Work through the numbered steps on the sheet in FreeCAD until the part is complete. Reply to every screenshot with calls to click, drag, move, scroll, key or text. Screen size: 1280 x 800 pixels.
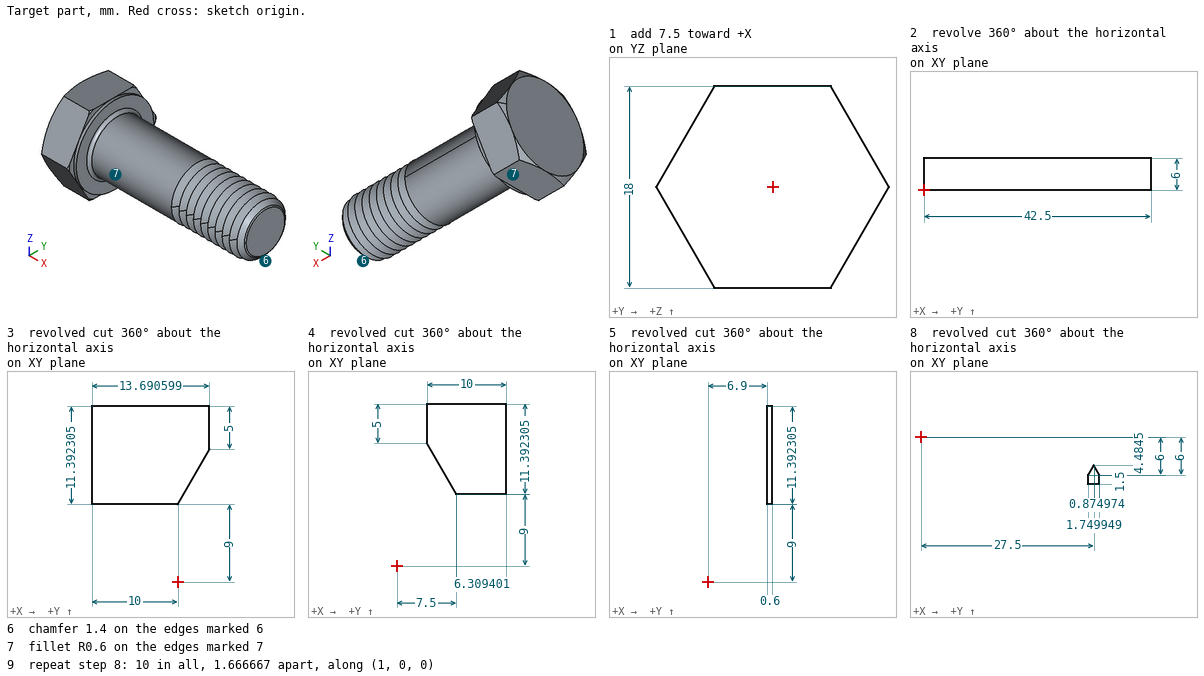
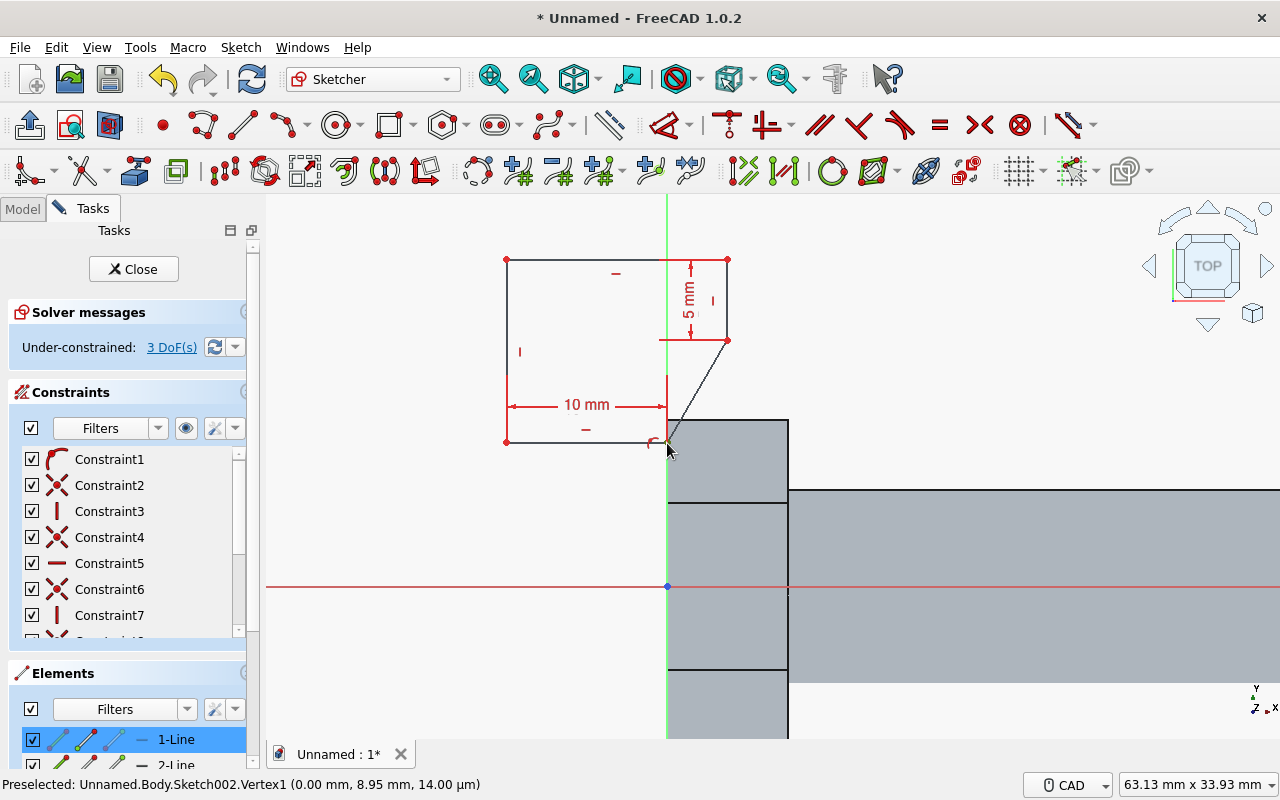
key(i)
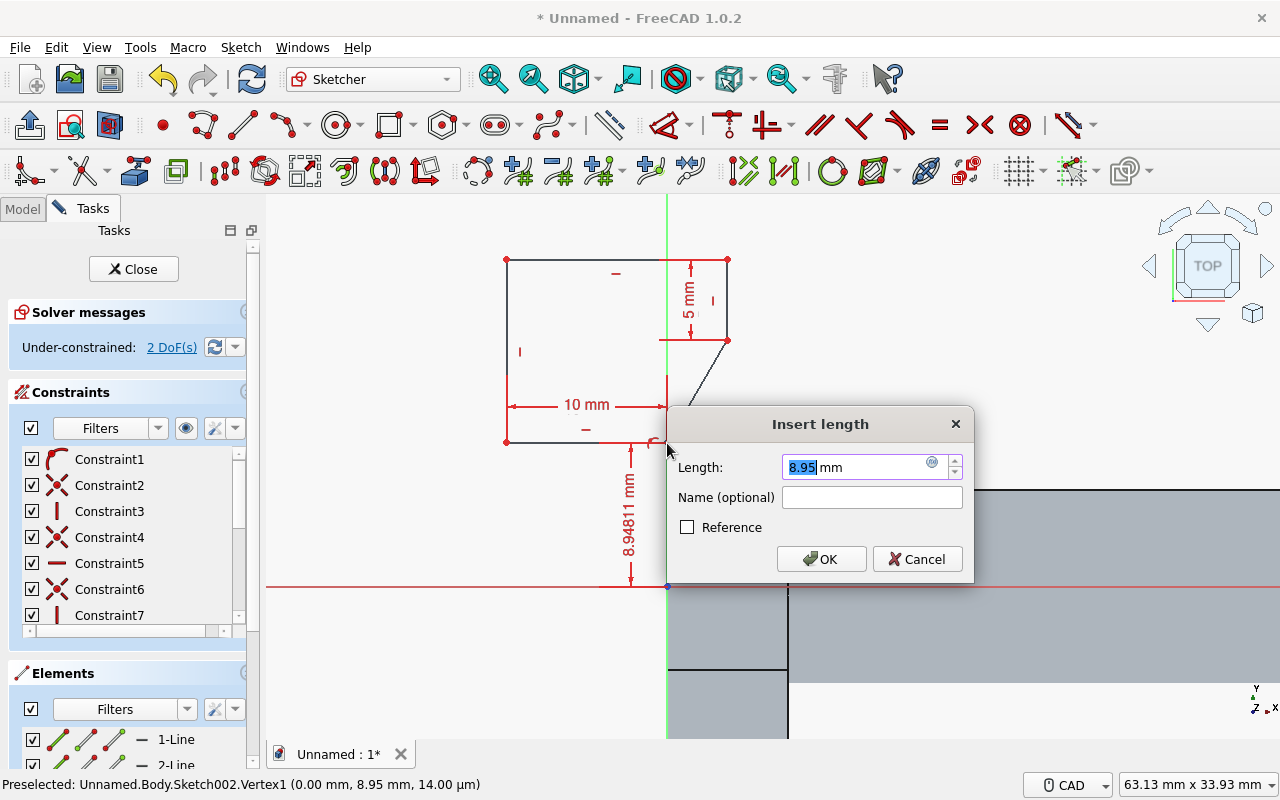
text(9)
key(Return)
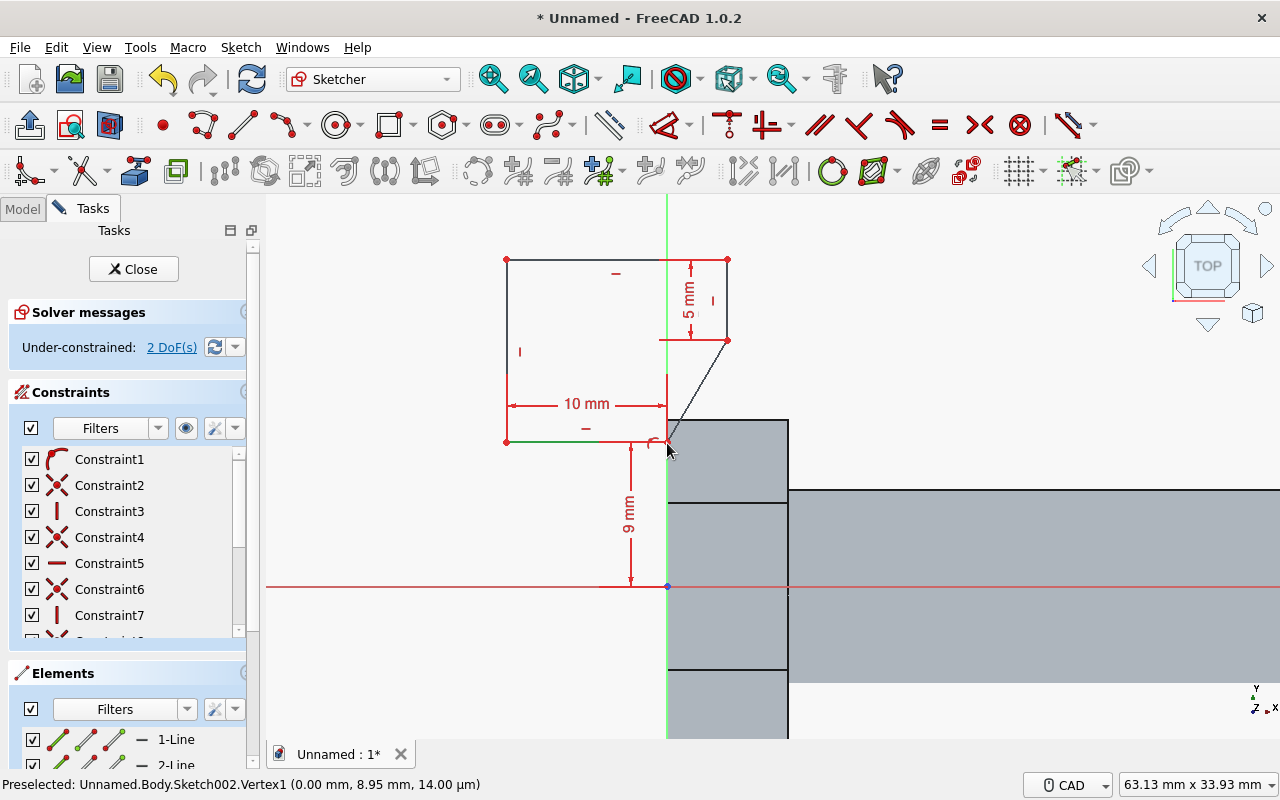
click(573, 260)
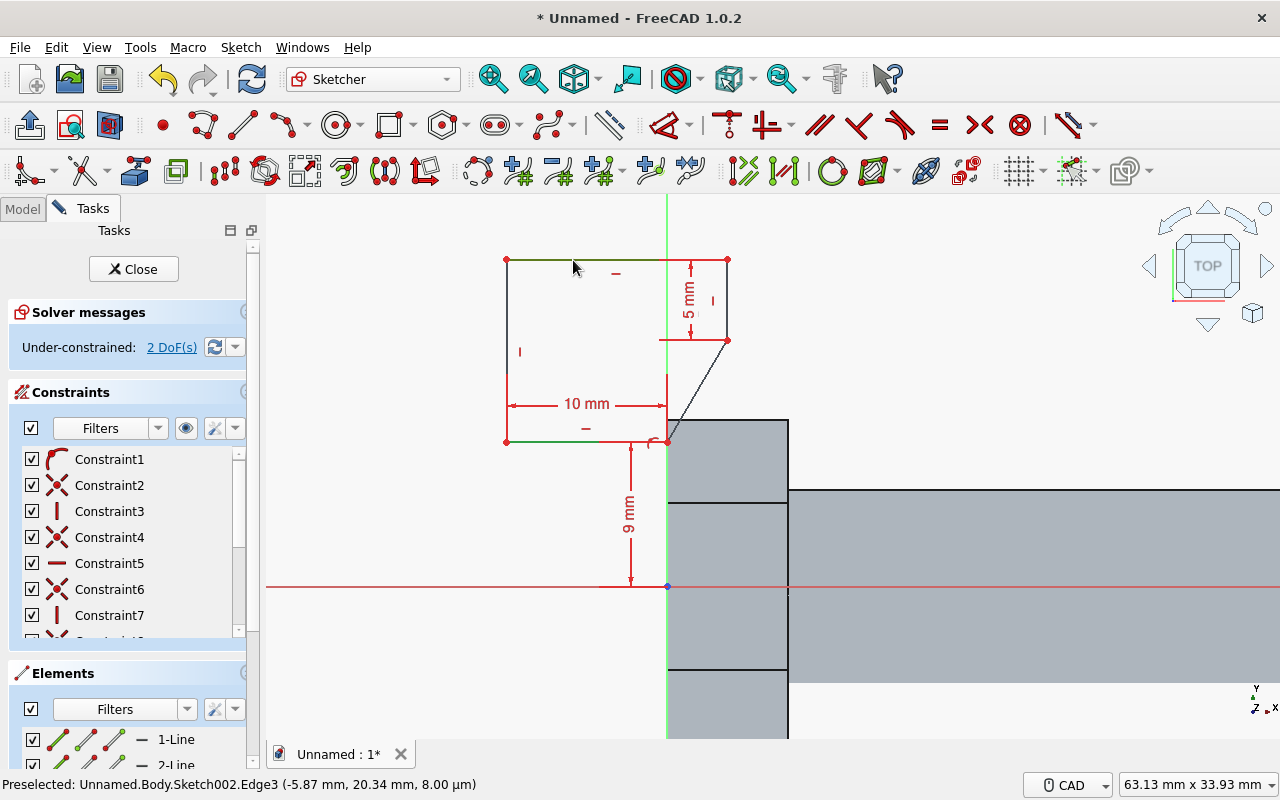
click(692, 126)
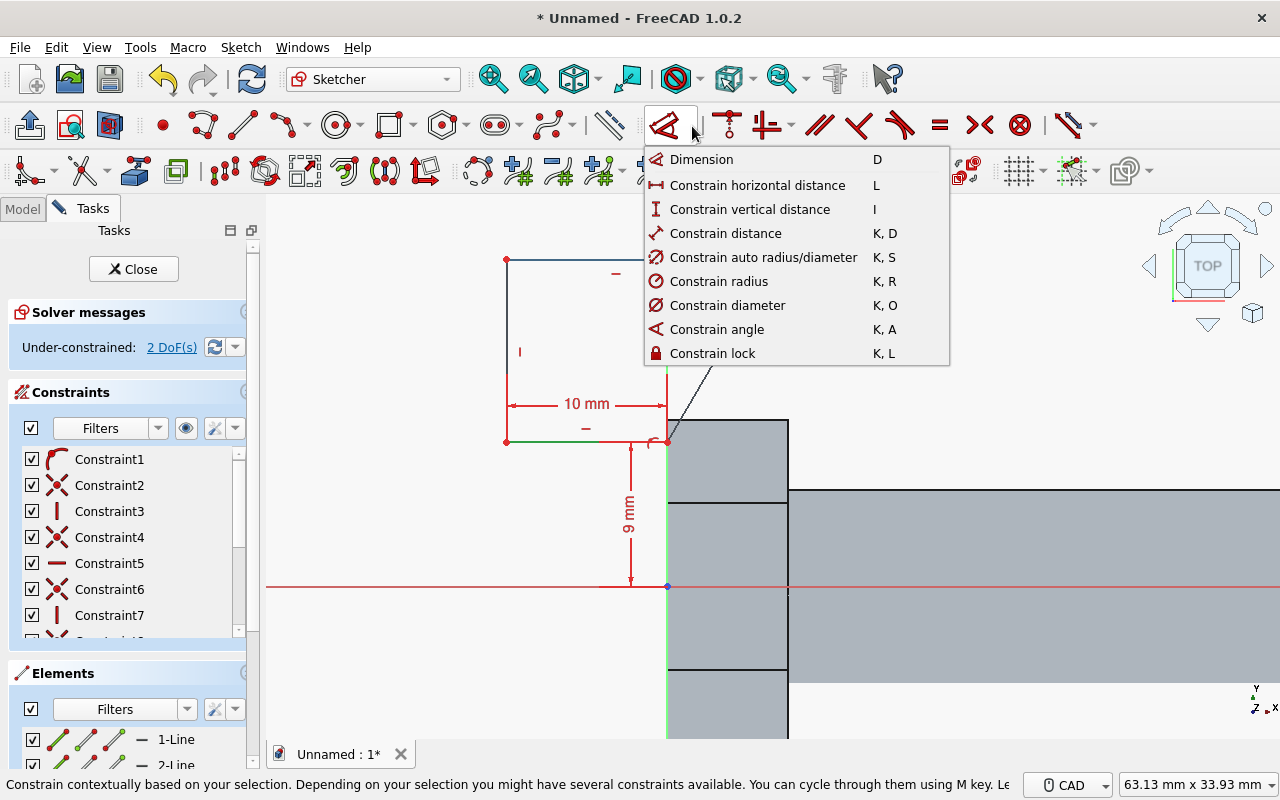
click(797, 185)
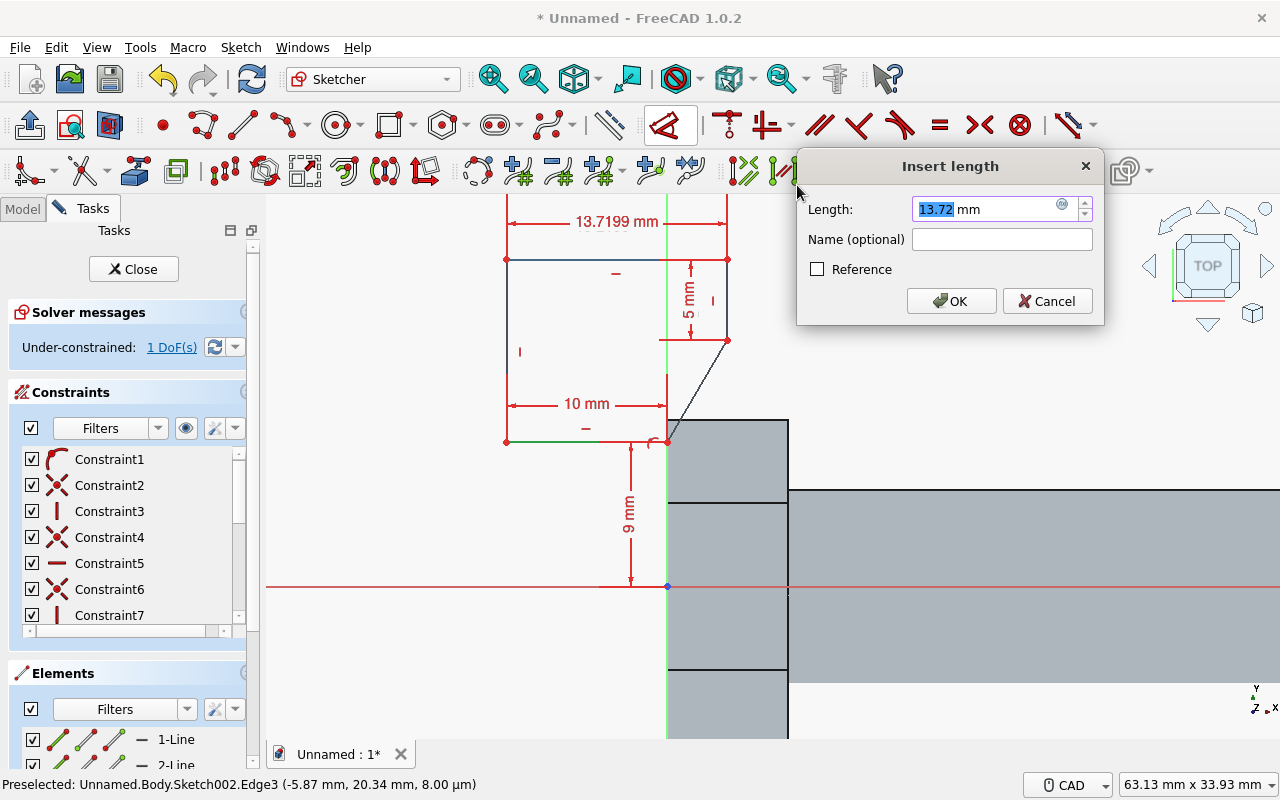
text(13.690599)
key(Return)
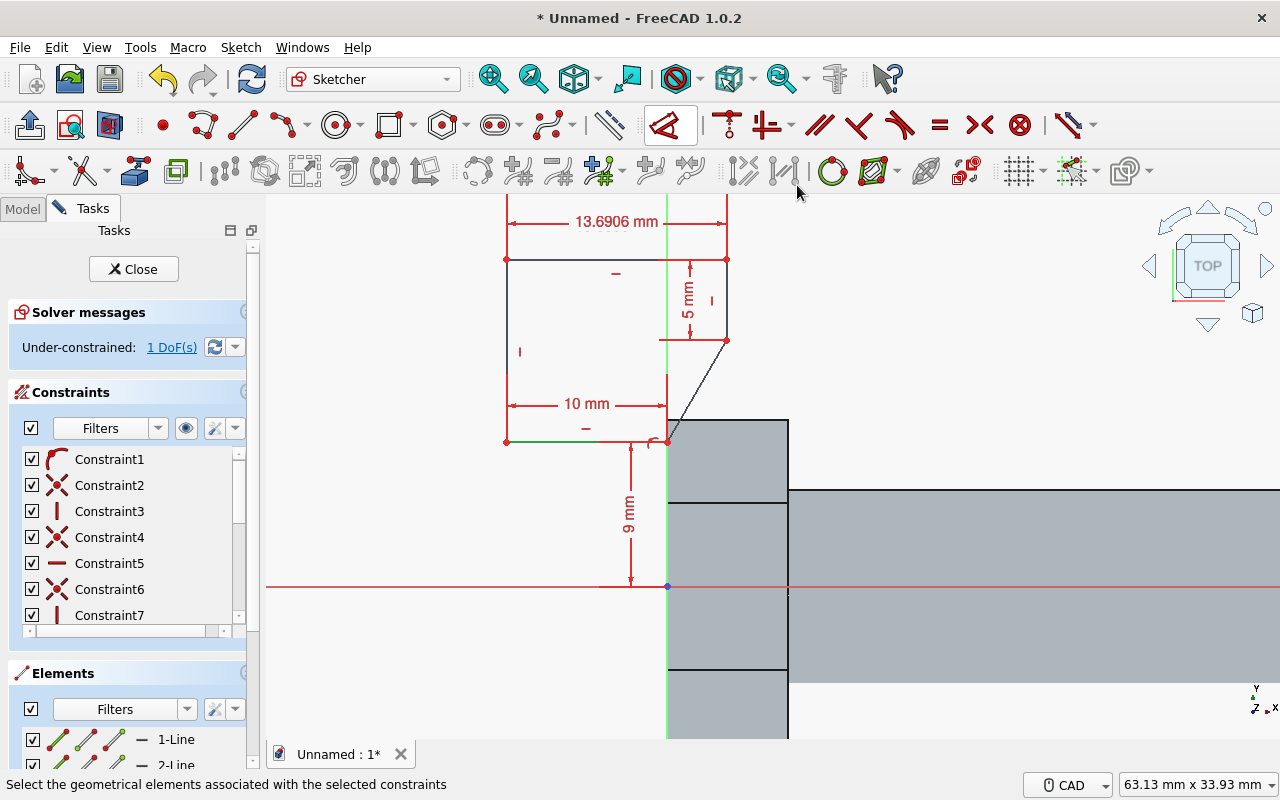
click(507, 315)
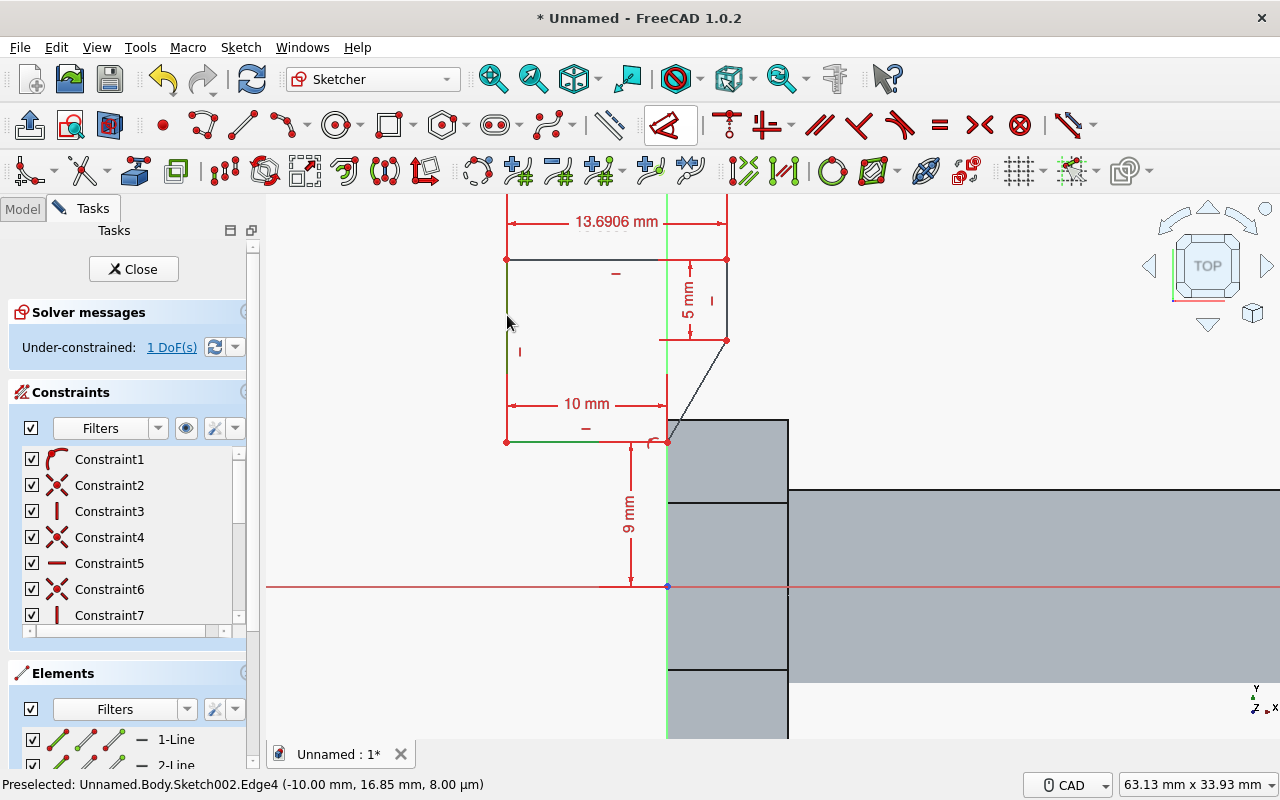
click(692, 126)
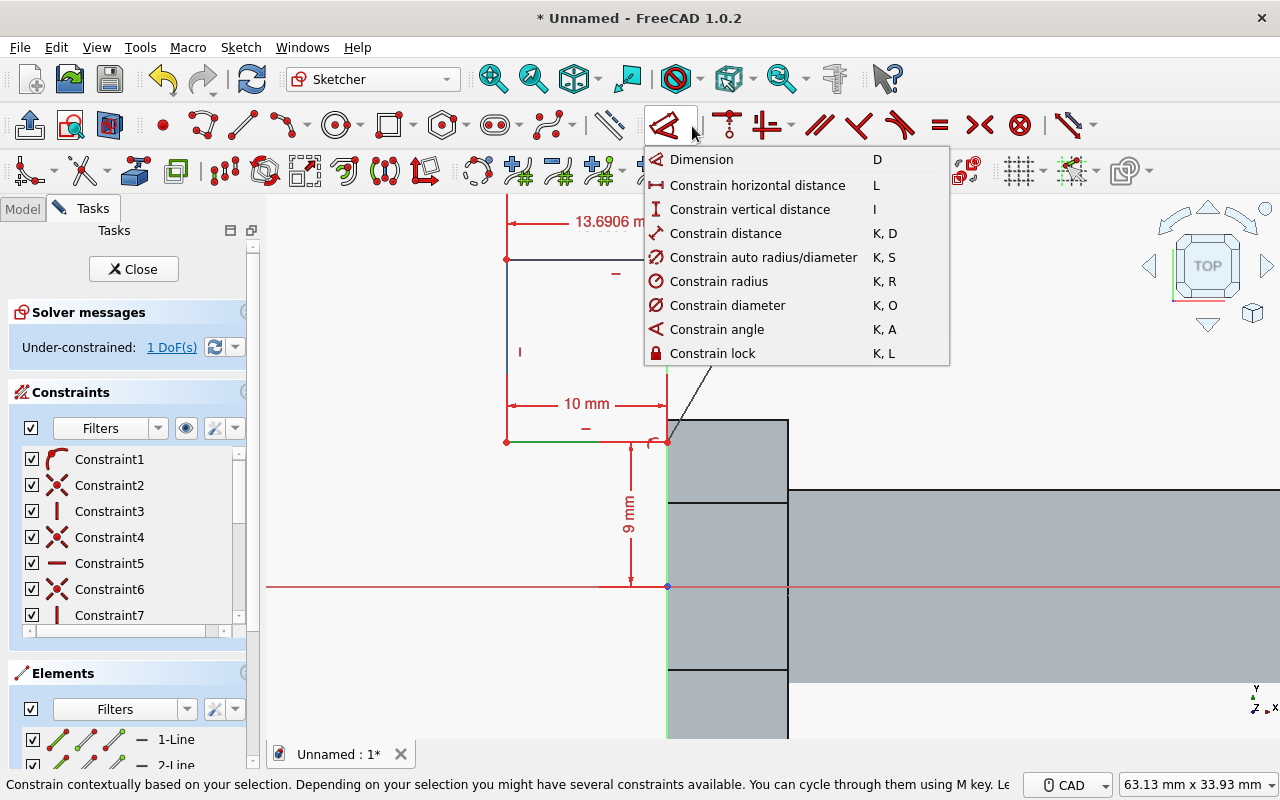
click(797, 209)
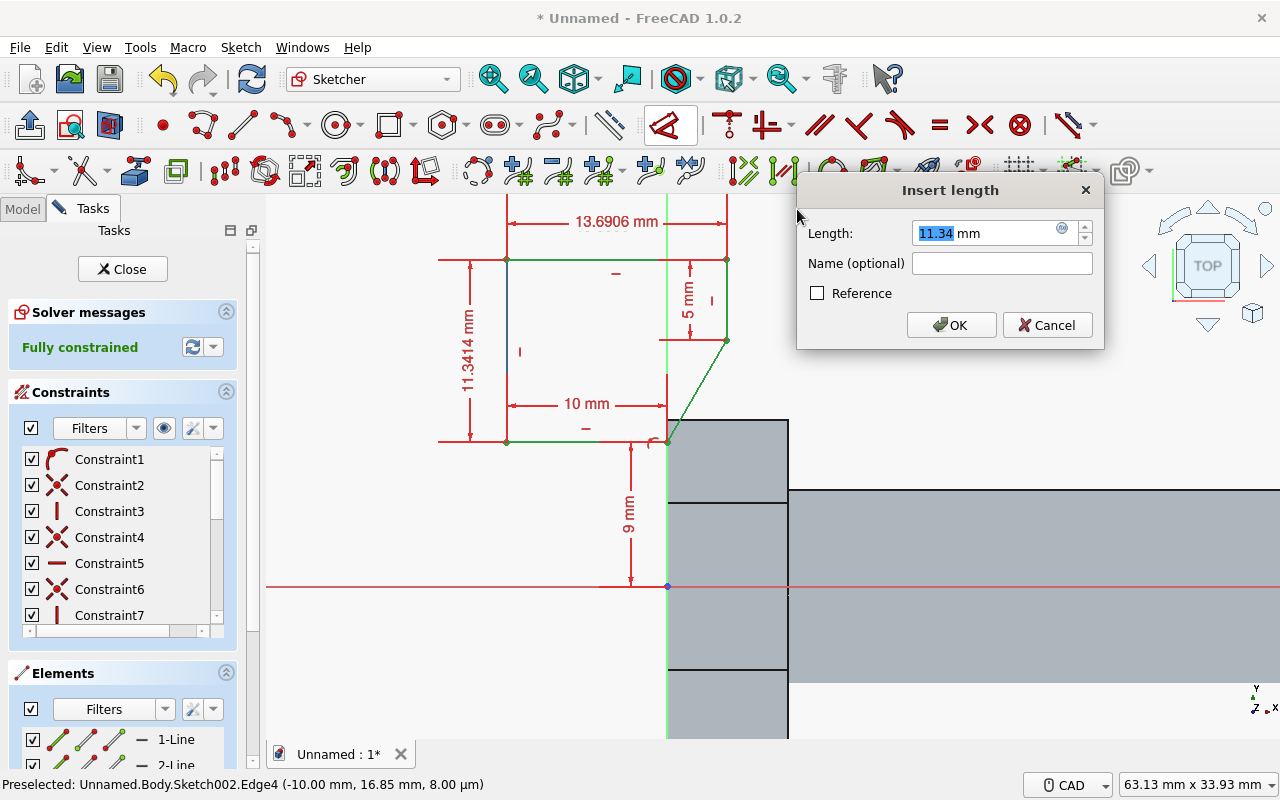
text(11.392305)
key(Return)